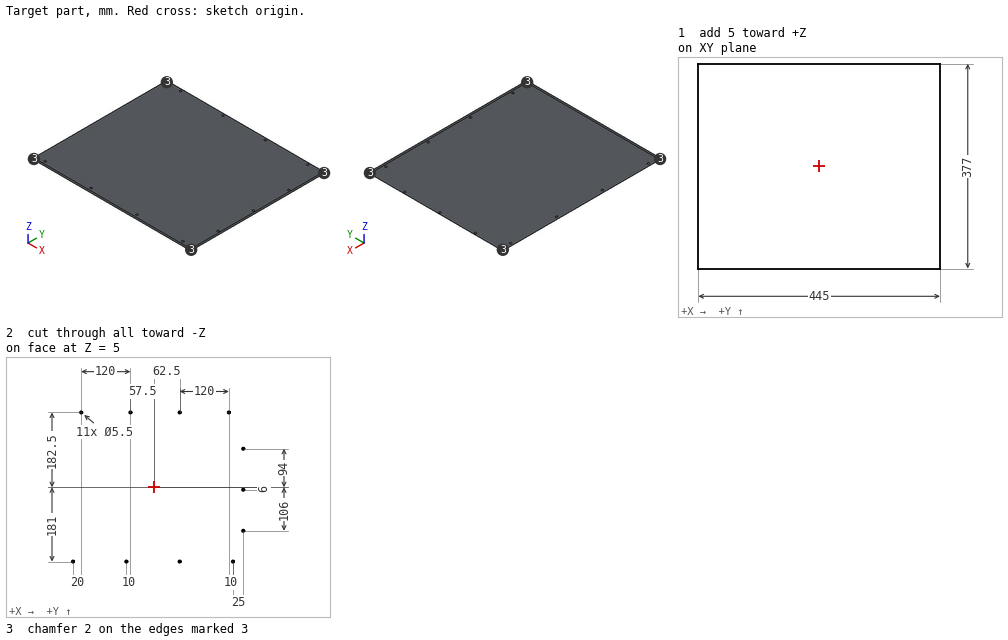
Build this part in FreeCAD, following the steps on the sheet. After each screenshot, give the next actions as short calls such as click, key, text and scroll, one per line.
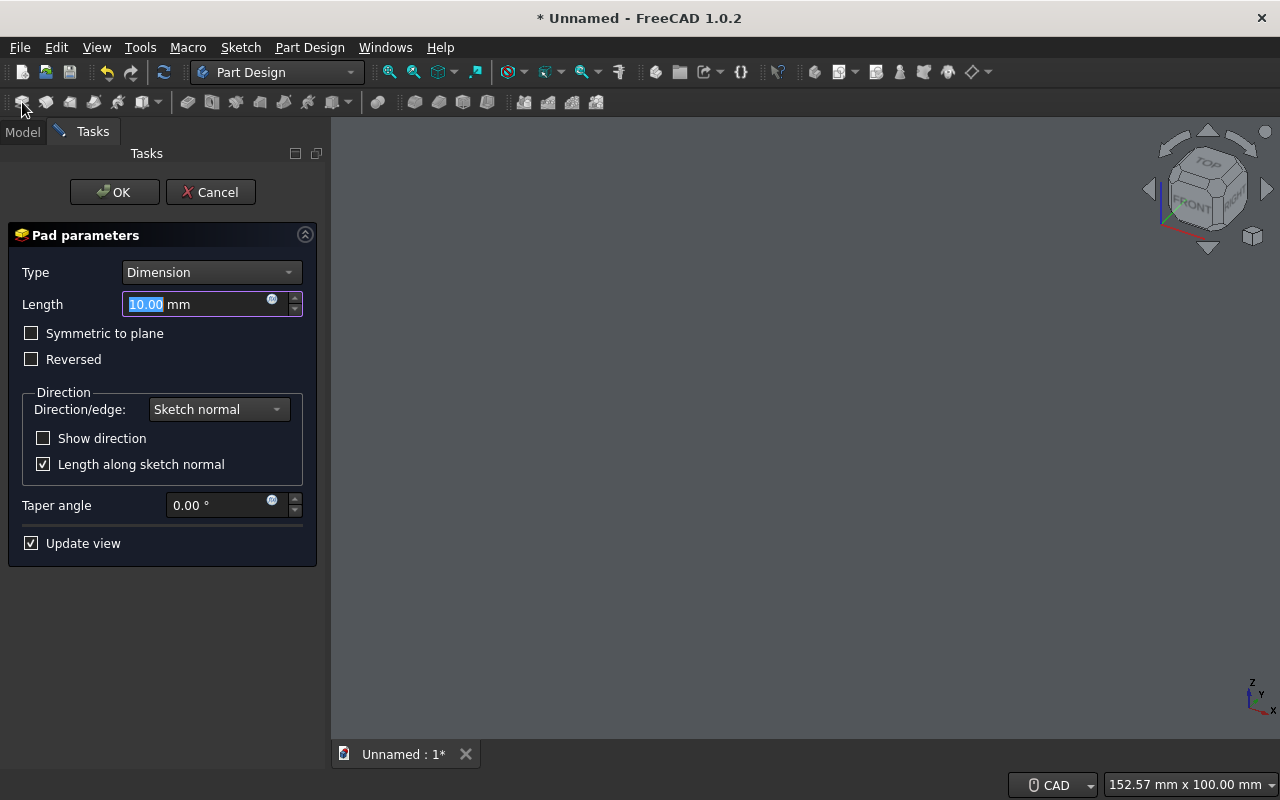
text(5)
key(Tab)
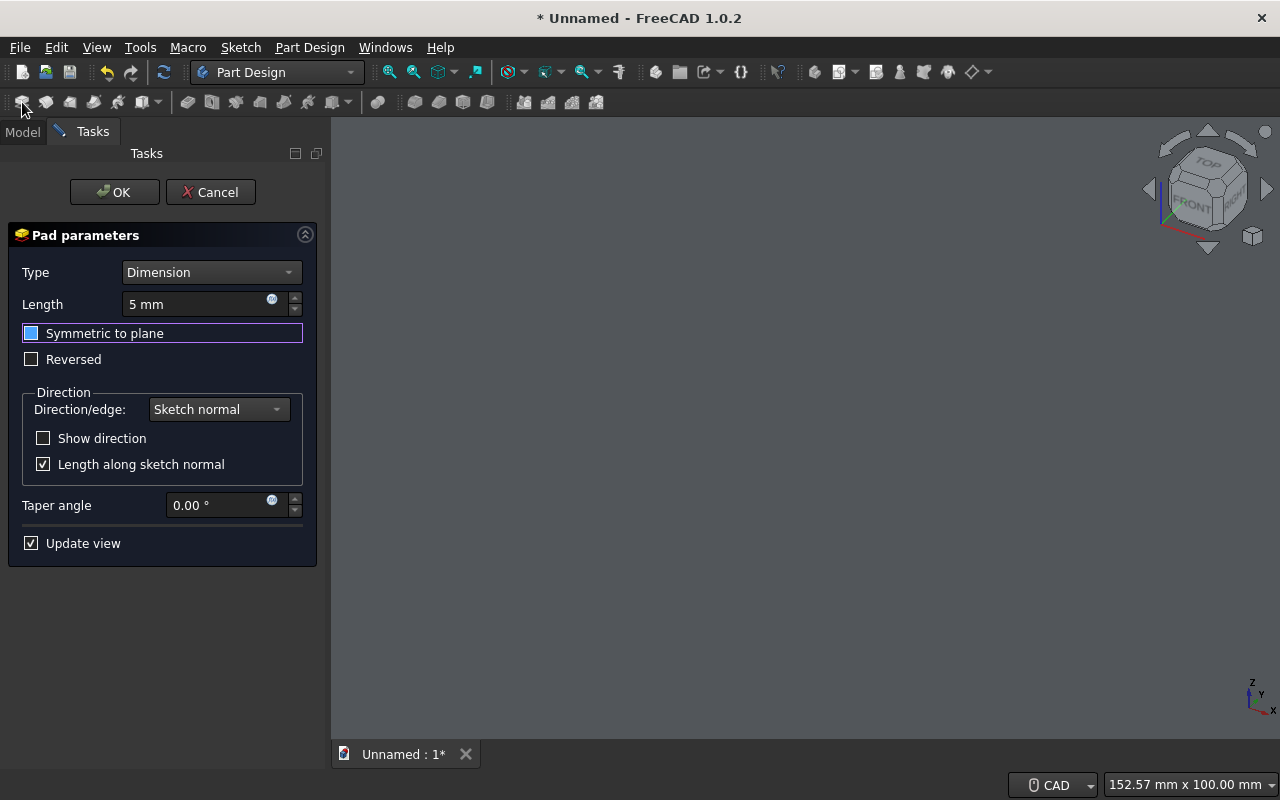
click(115, 192)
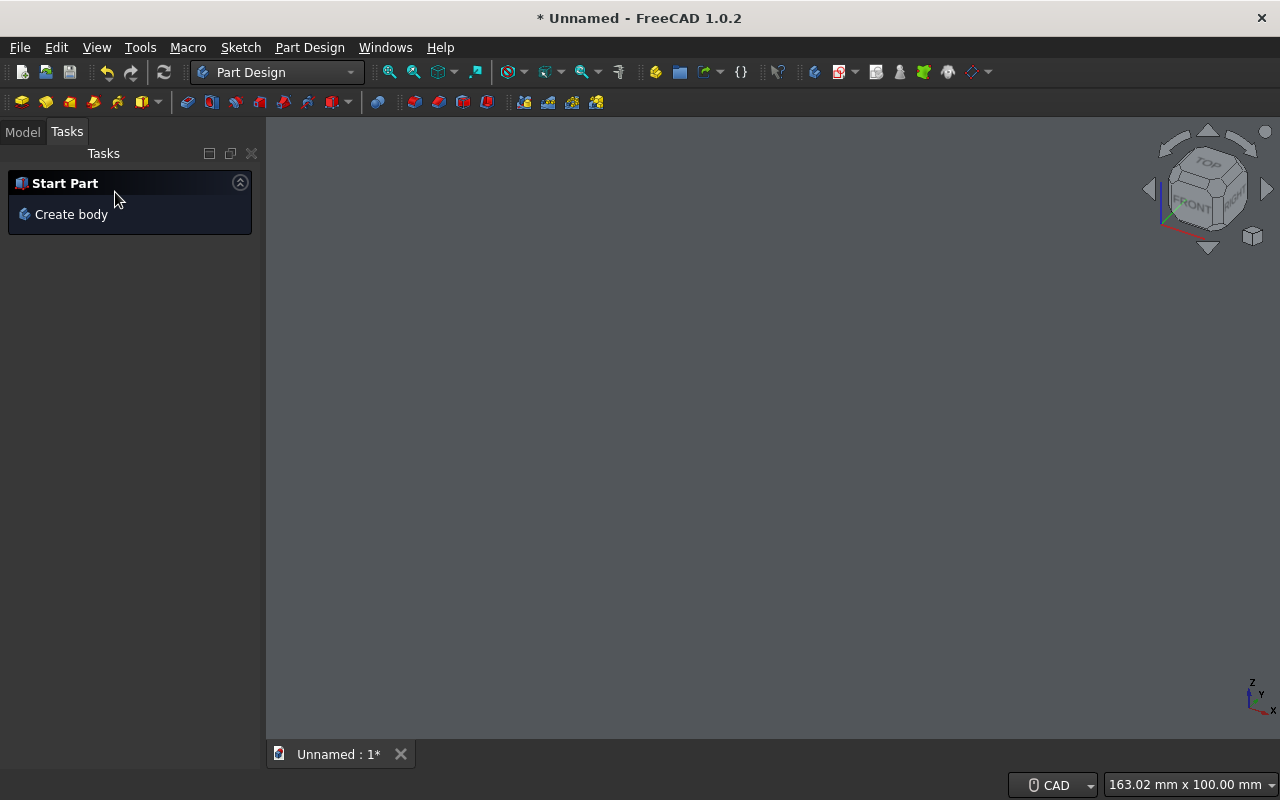
key(v)
key(f)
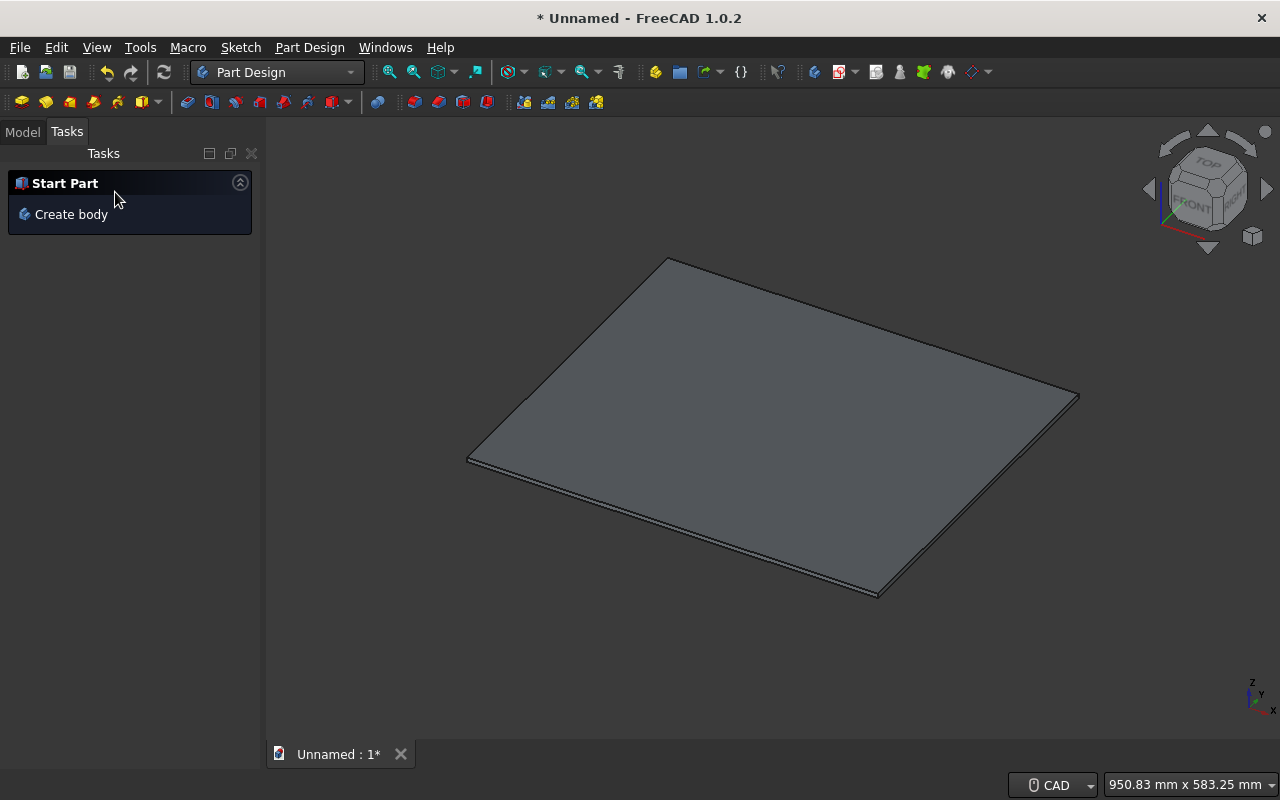
click(773, 425)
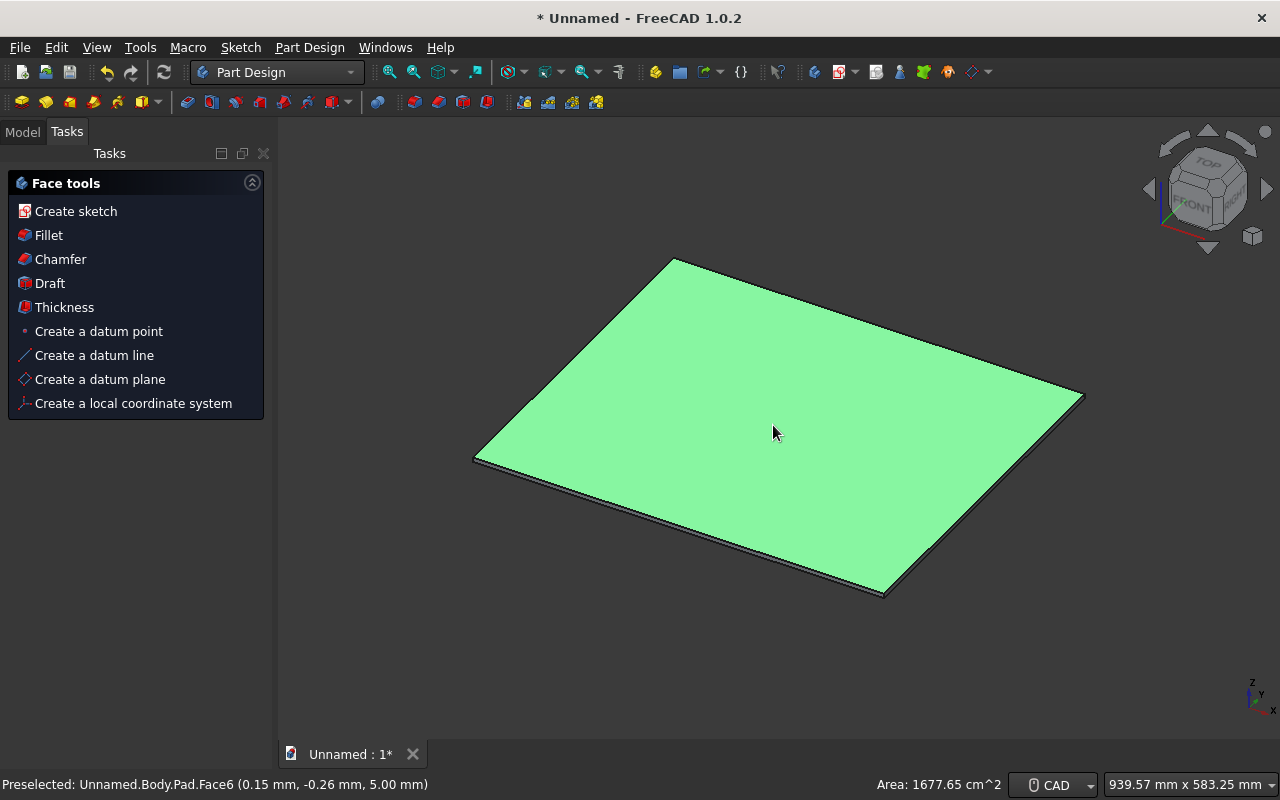
click(840, 72)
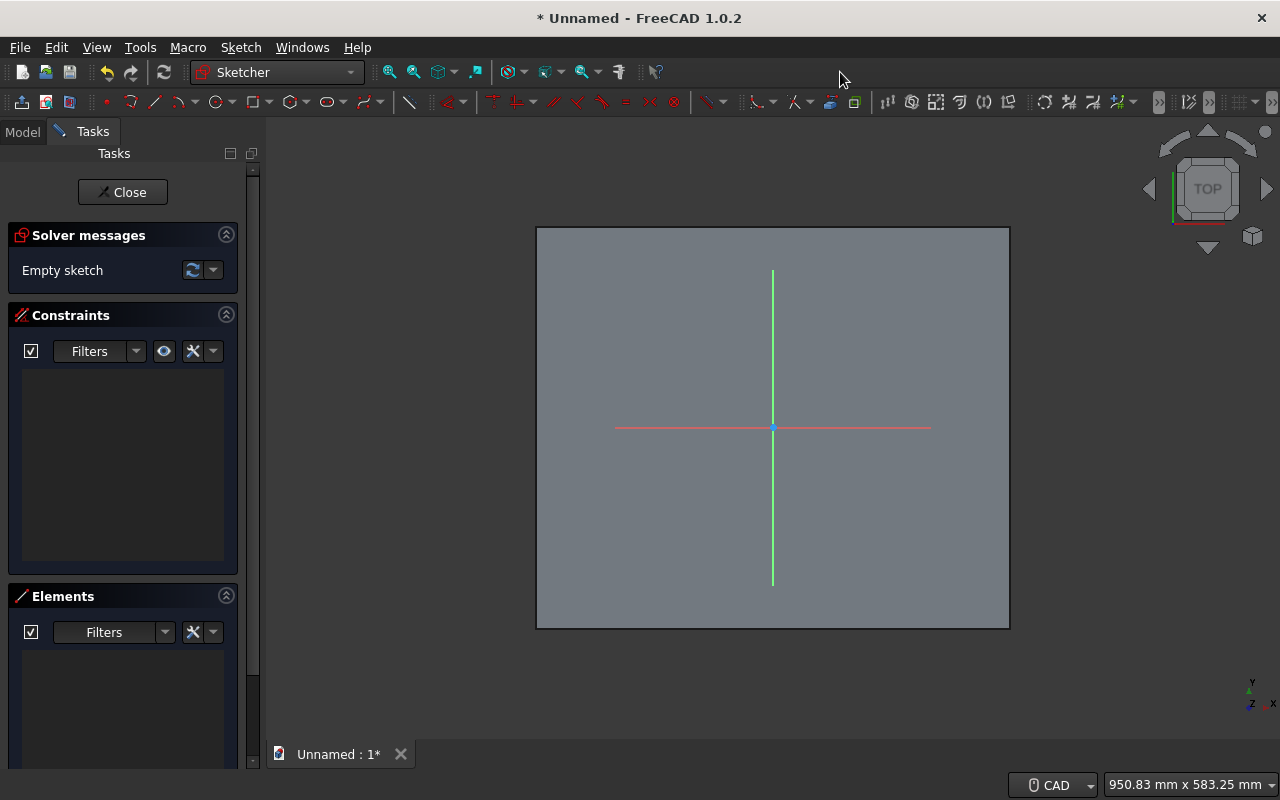
click(216, 102)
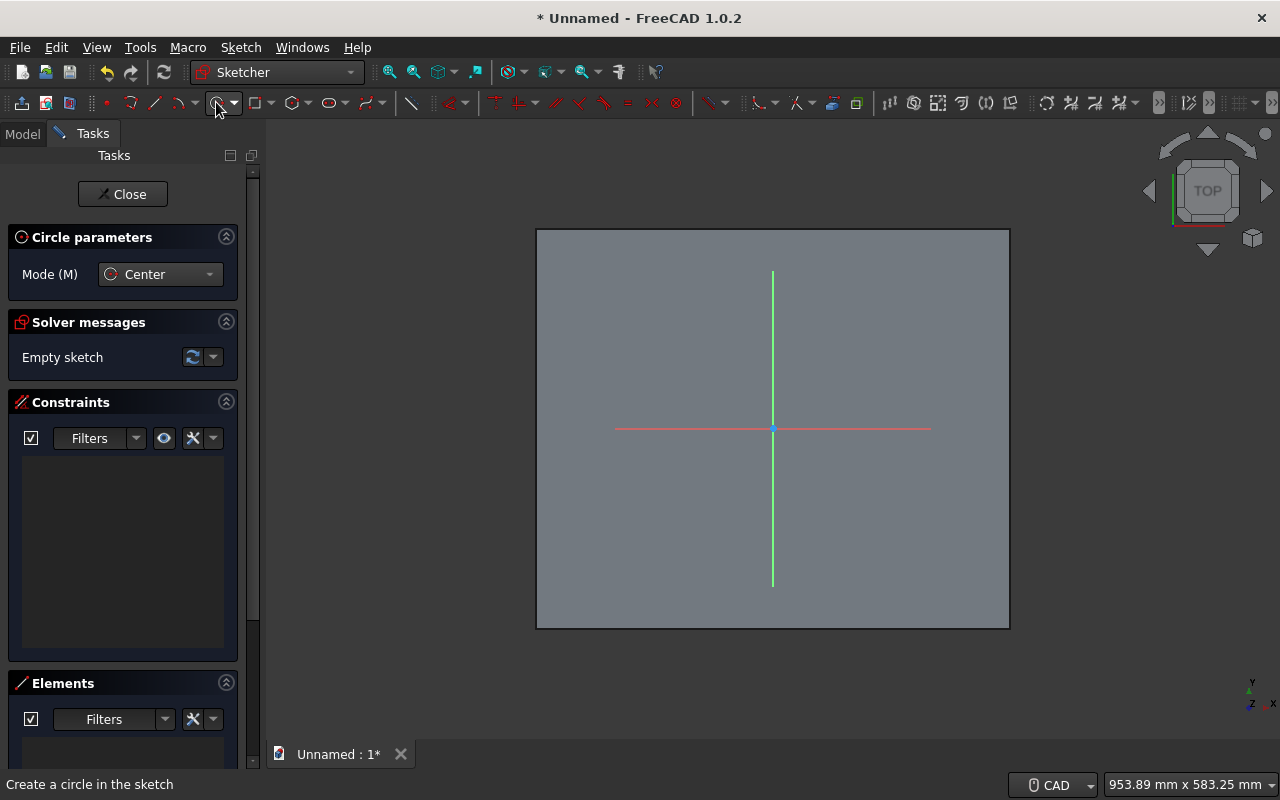
scroll(584, 235, up, 11)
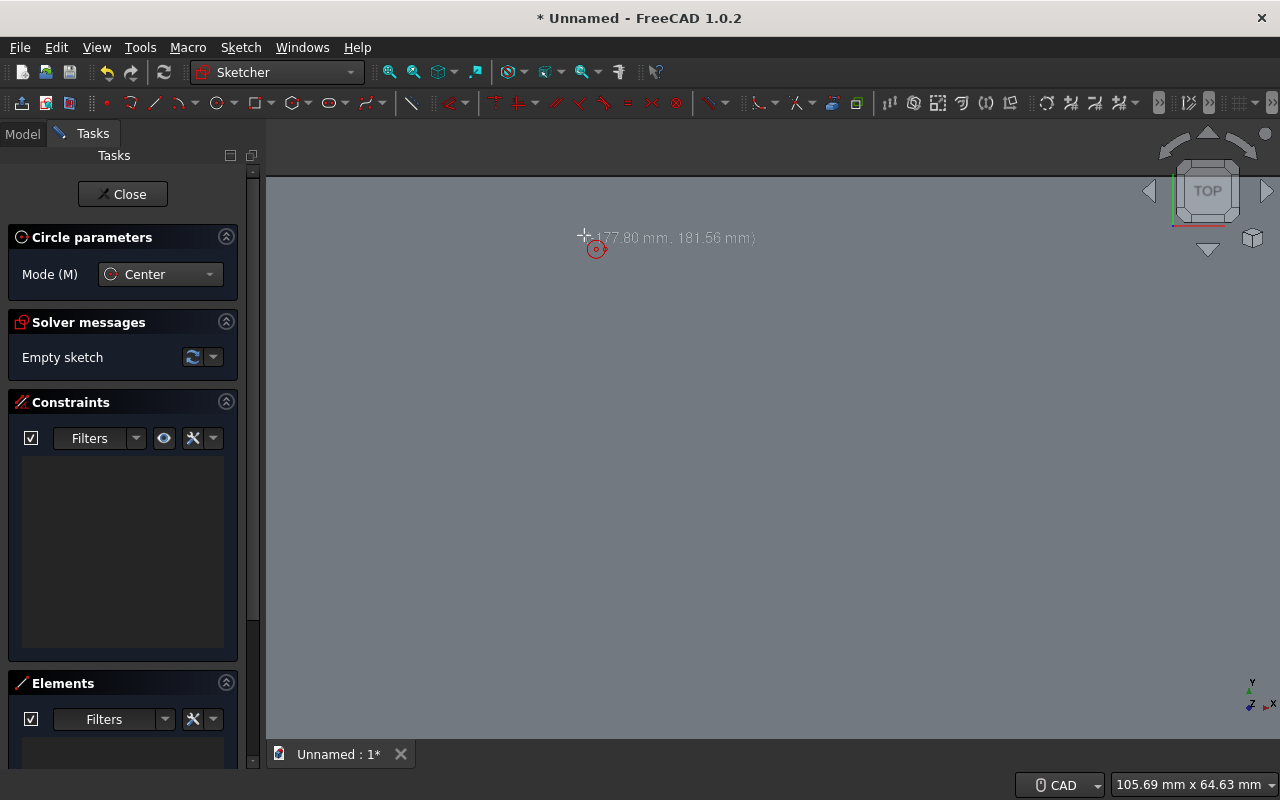
scroll(495, 236, down, 11)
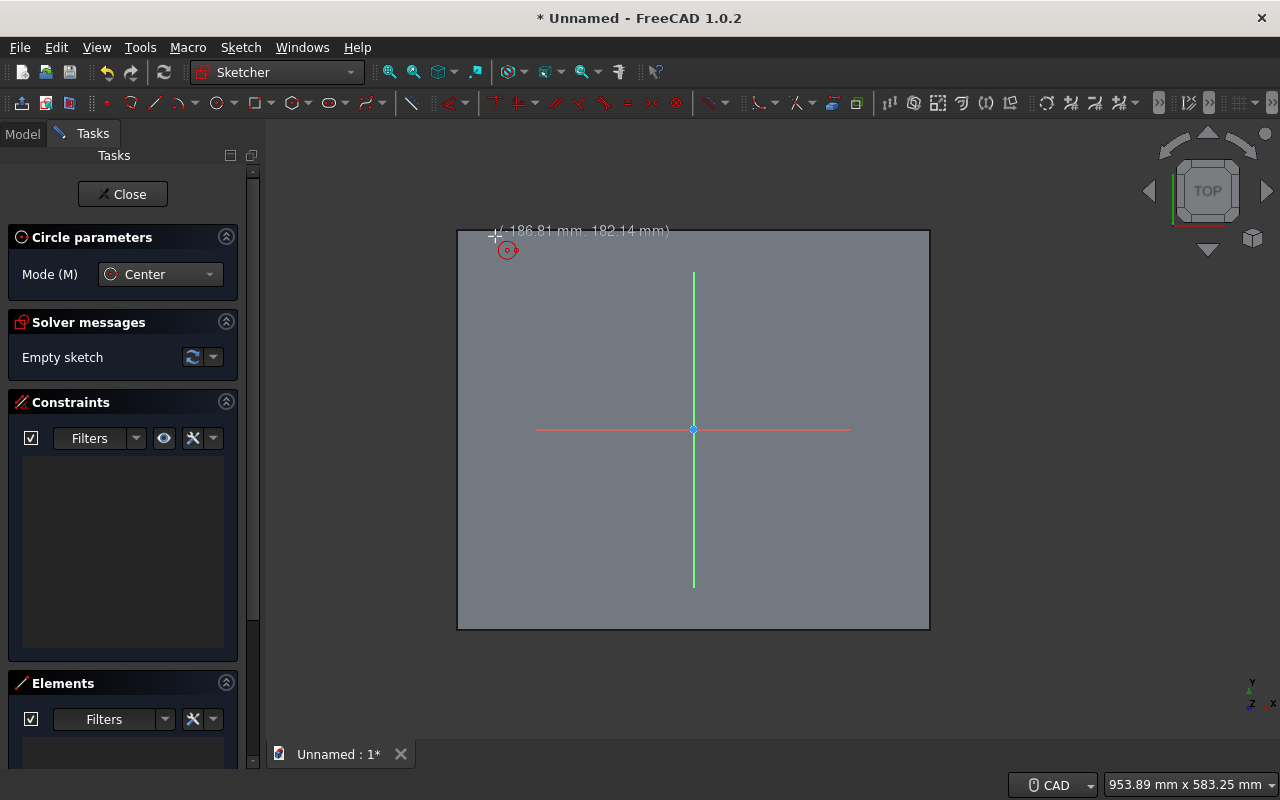
click(505, 236)
move(507, 234)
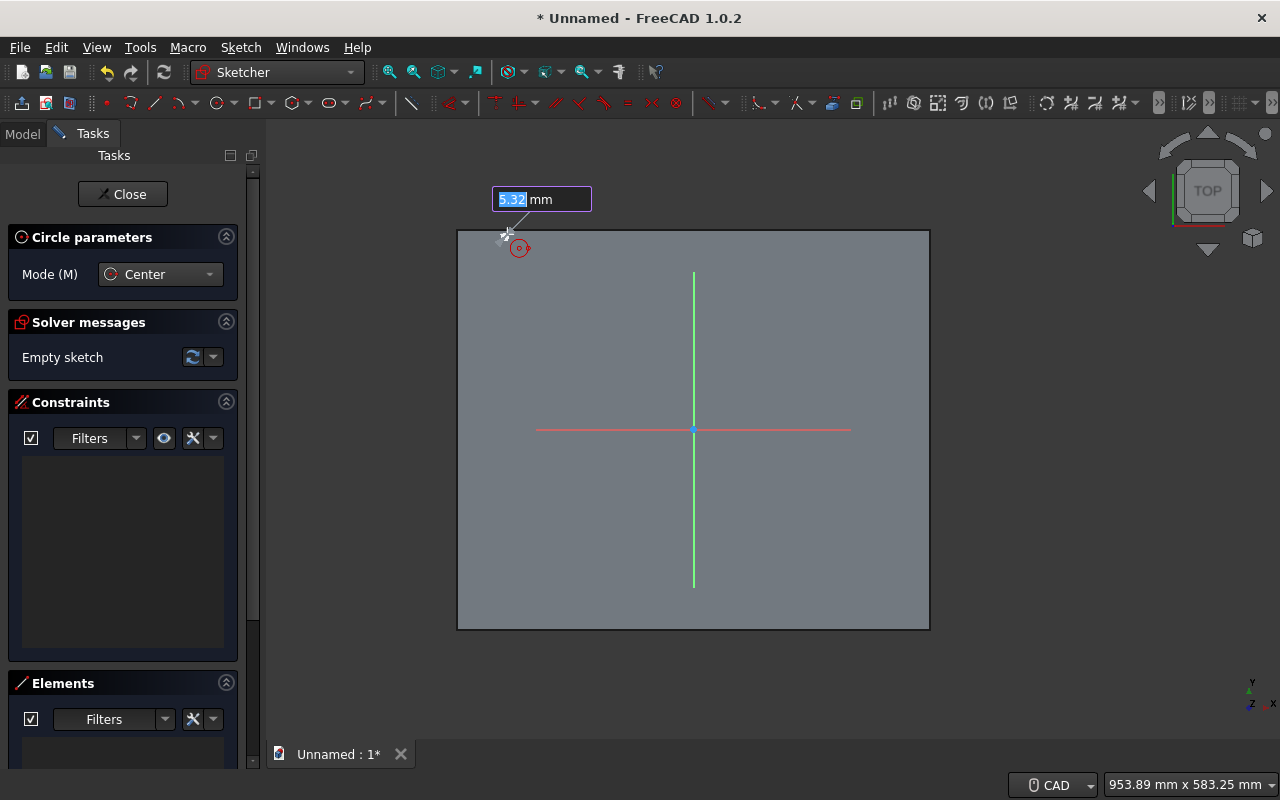
text(5.5)
key(Return)